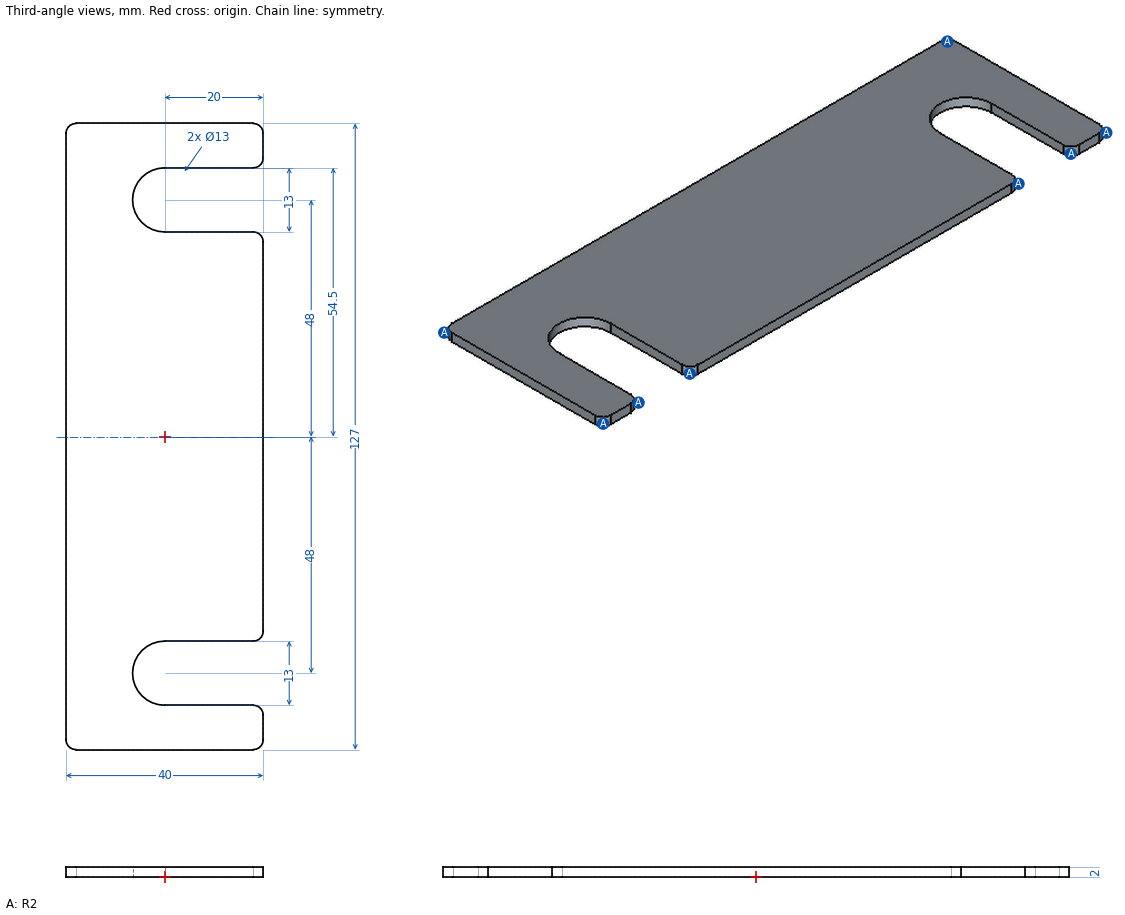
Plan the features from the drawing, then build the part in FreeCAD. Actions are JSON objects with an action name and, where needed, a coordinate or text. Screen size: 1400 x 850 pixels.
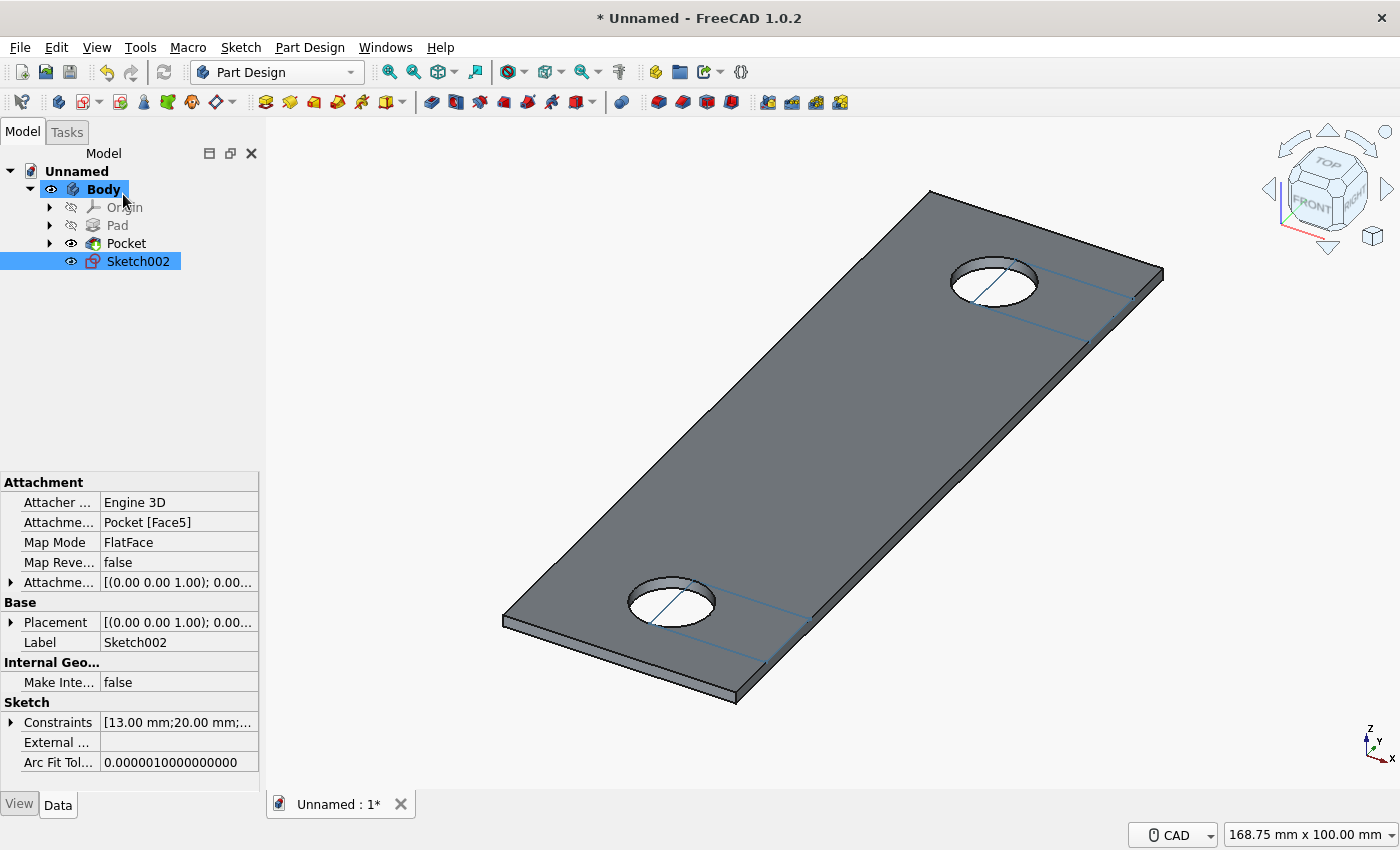
{"action": "left_click", "coordinate": [432, 102]}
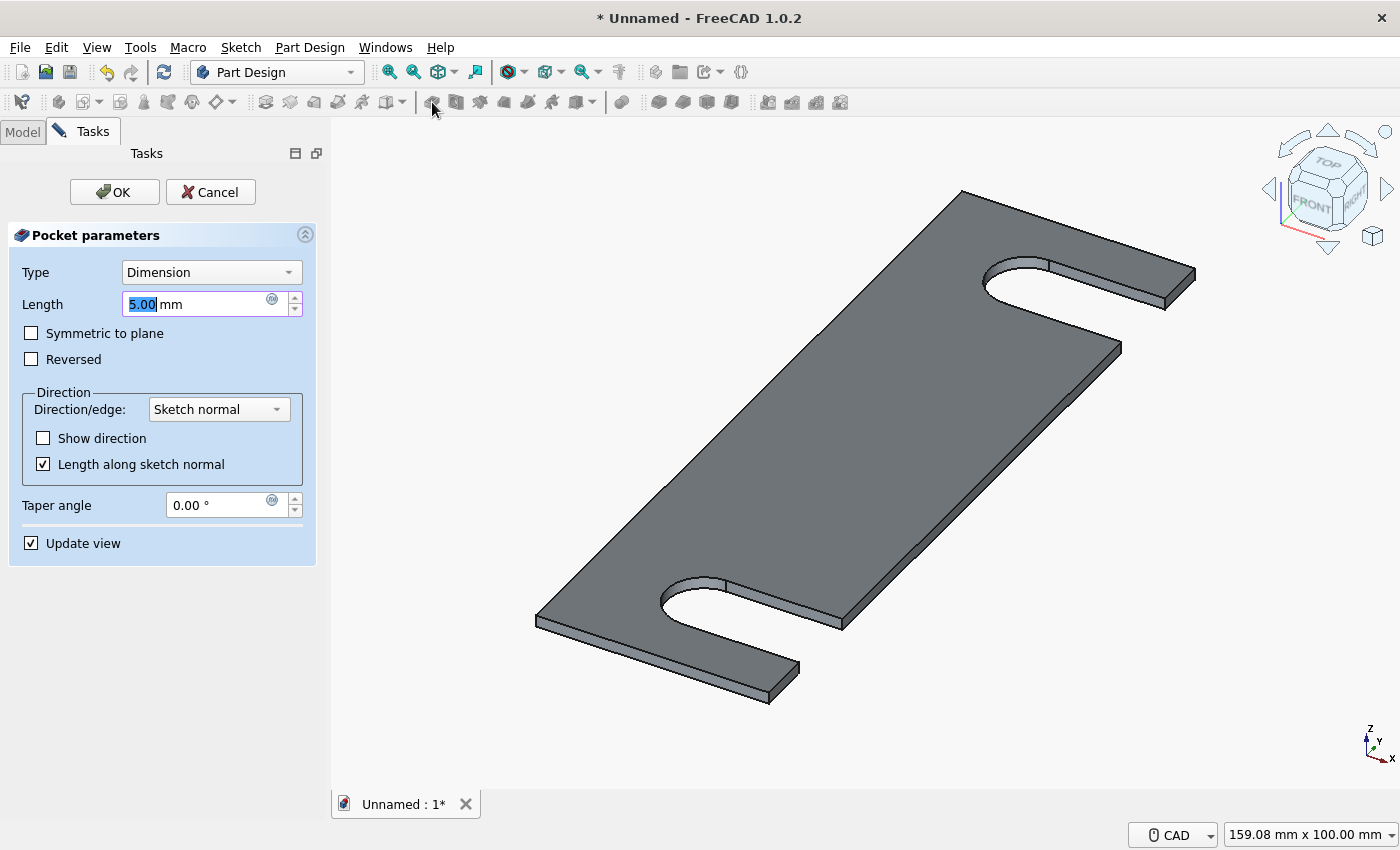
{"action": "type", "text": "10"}
{"action": "key", "text": "Tab"}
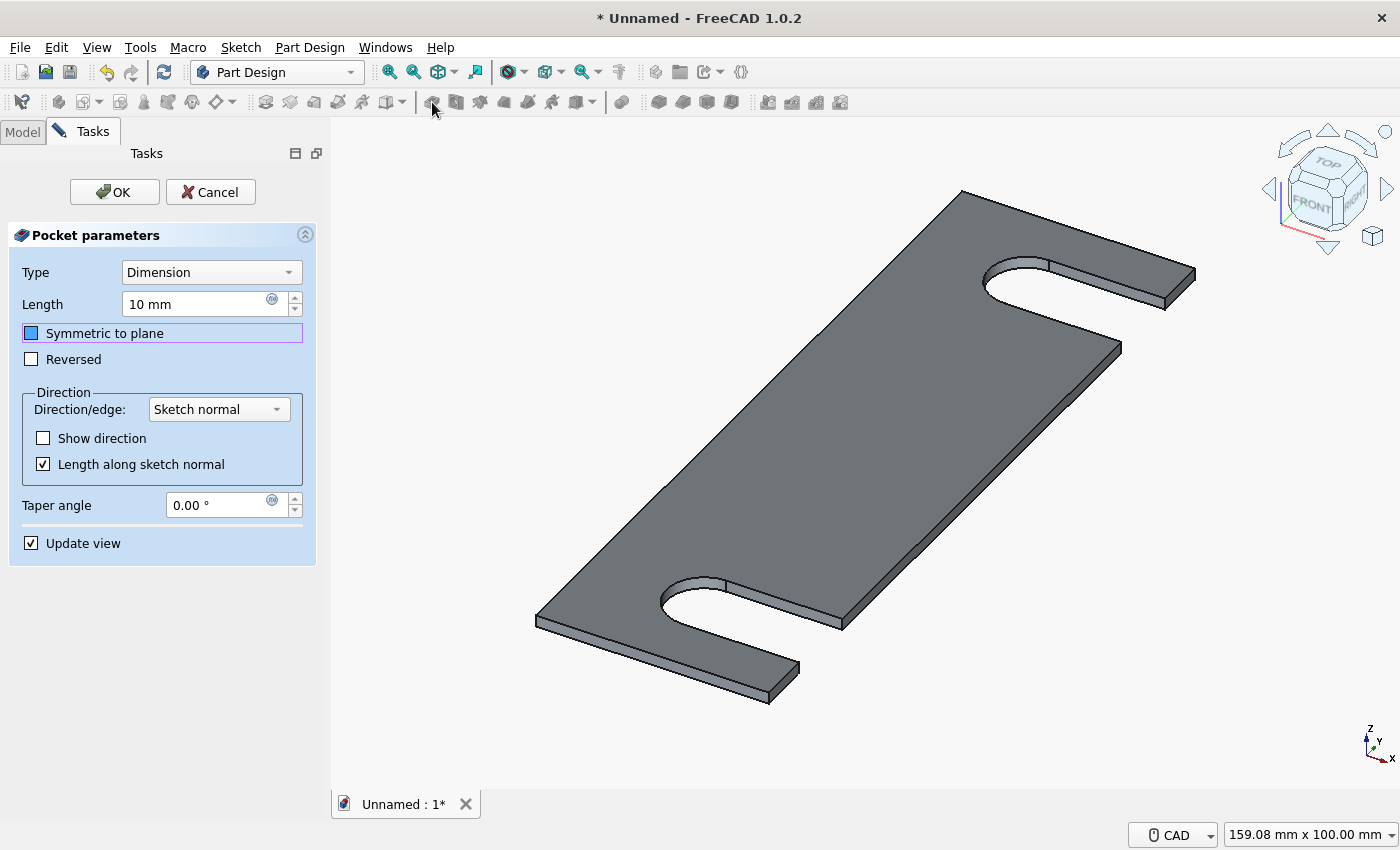
{"action": "left_click", "coordinate": [115, 192]}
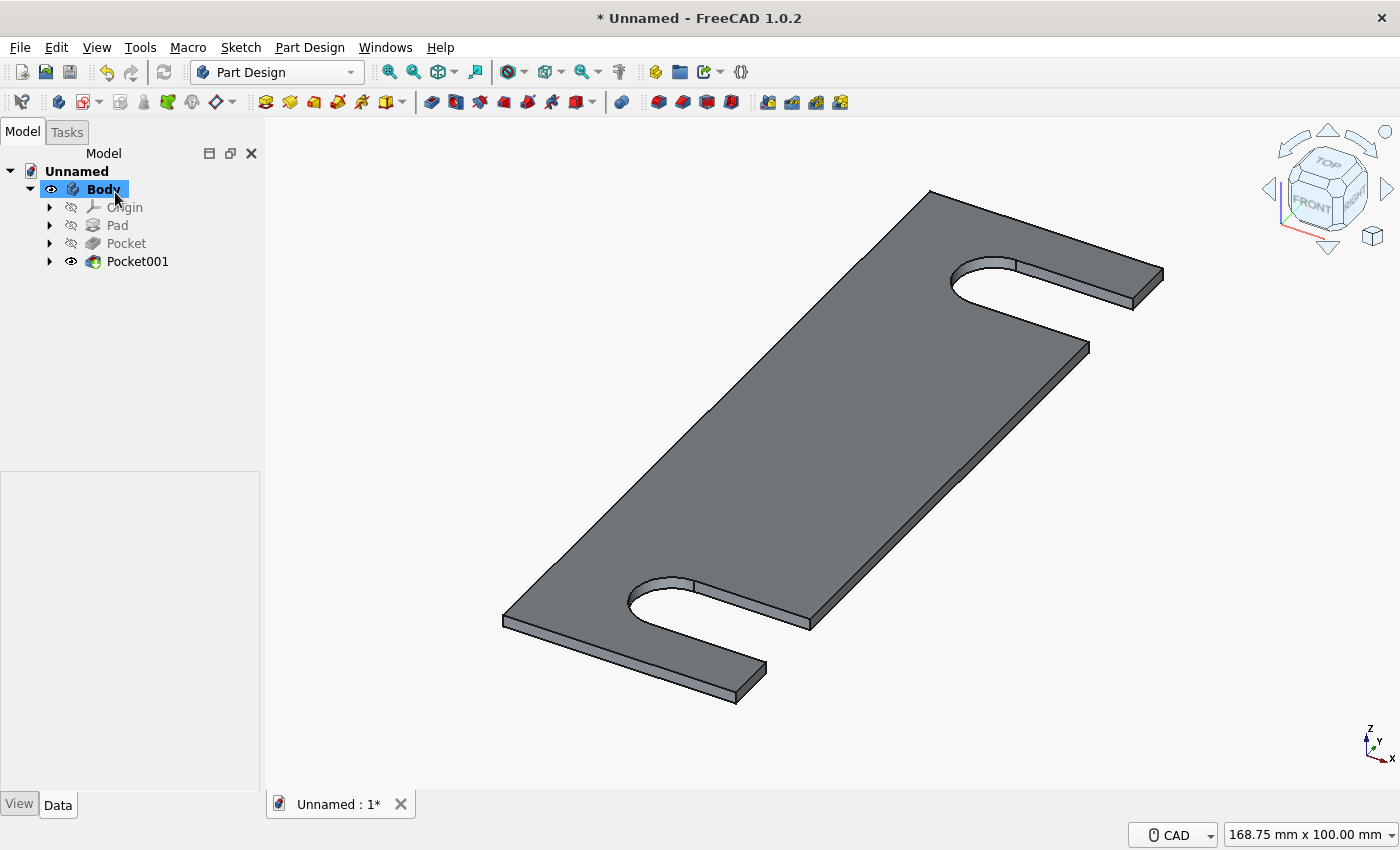
{"action": "left_click", "coordinate": [1133, 304]}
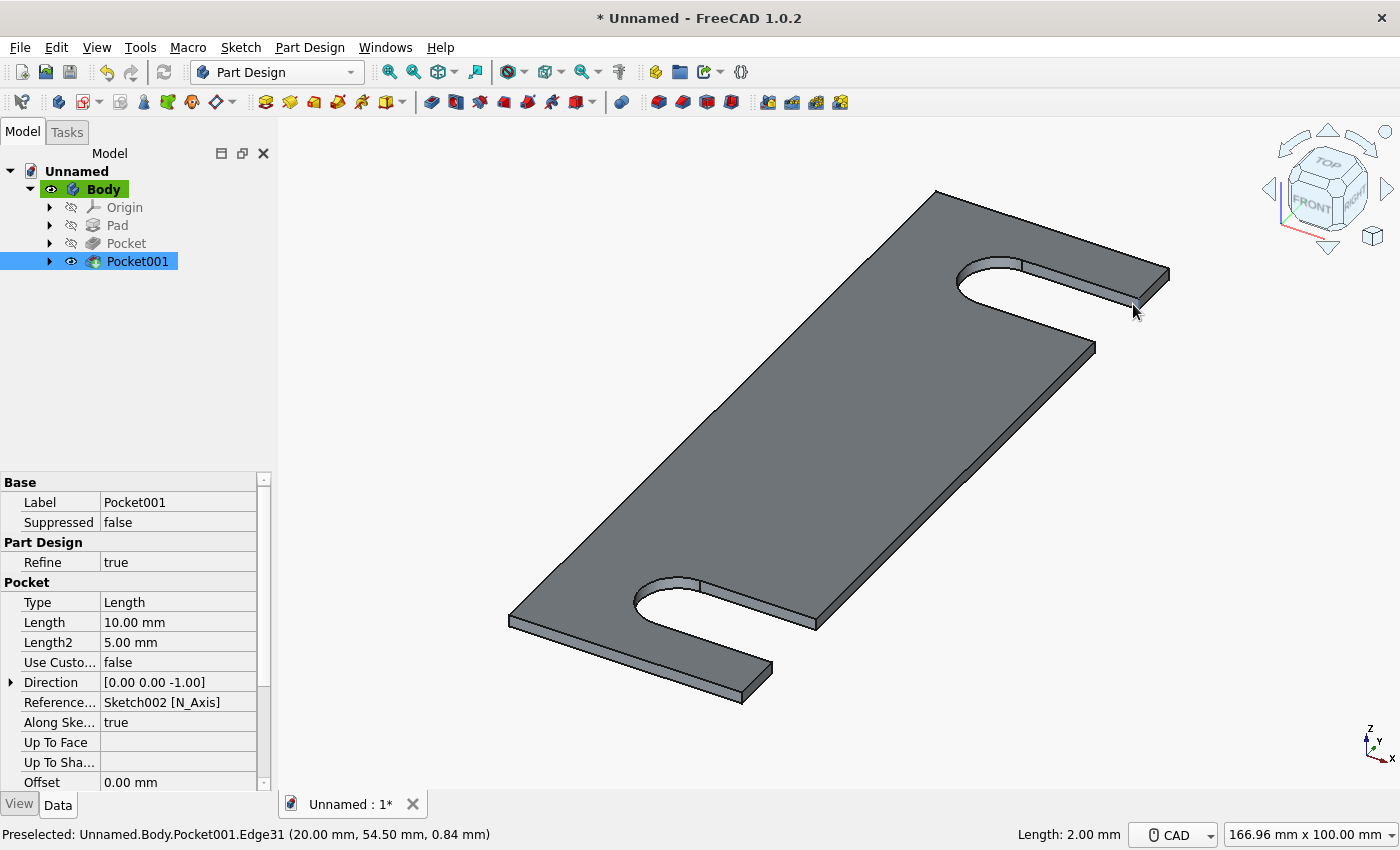
{"action": "left_click", "coordinate": [816, 624], "text": "ctrl"}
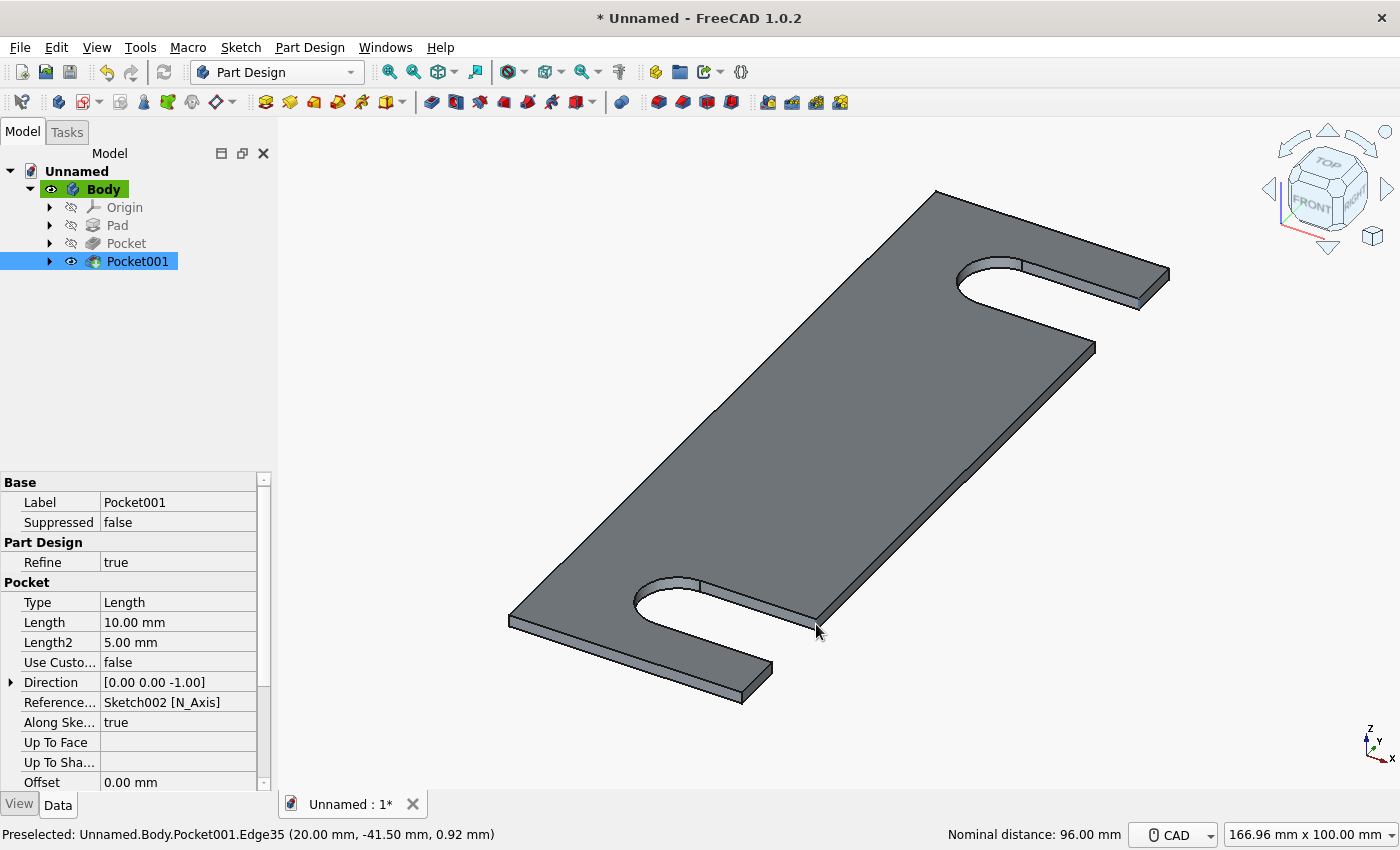
{"action": "left_click", "coordinate": [742, 698], "text": "ctrl"}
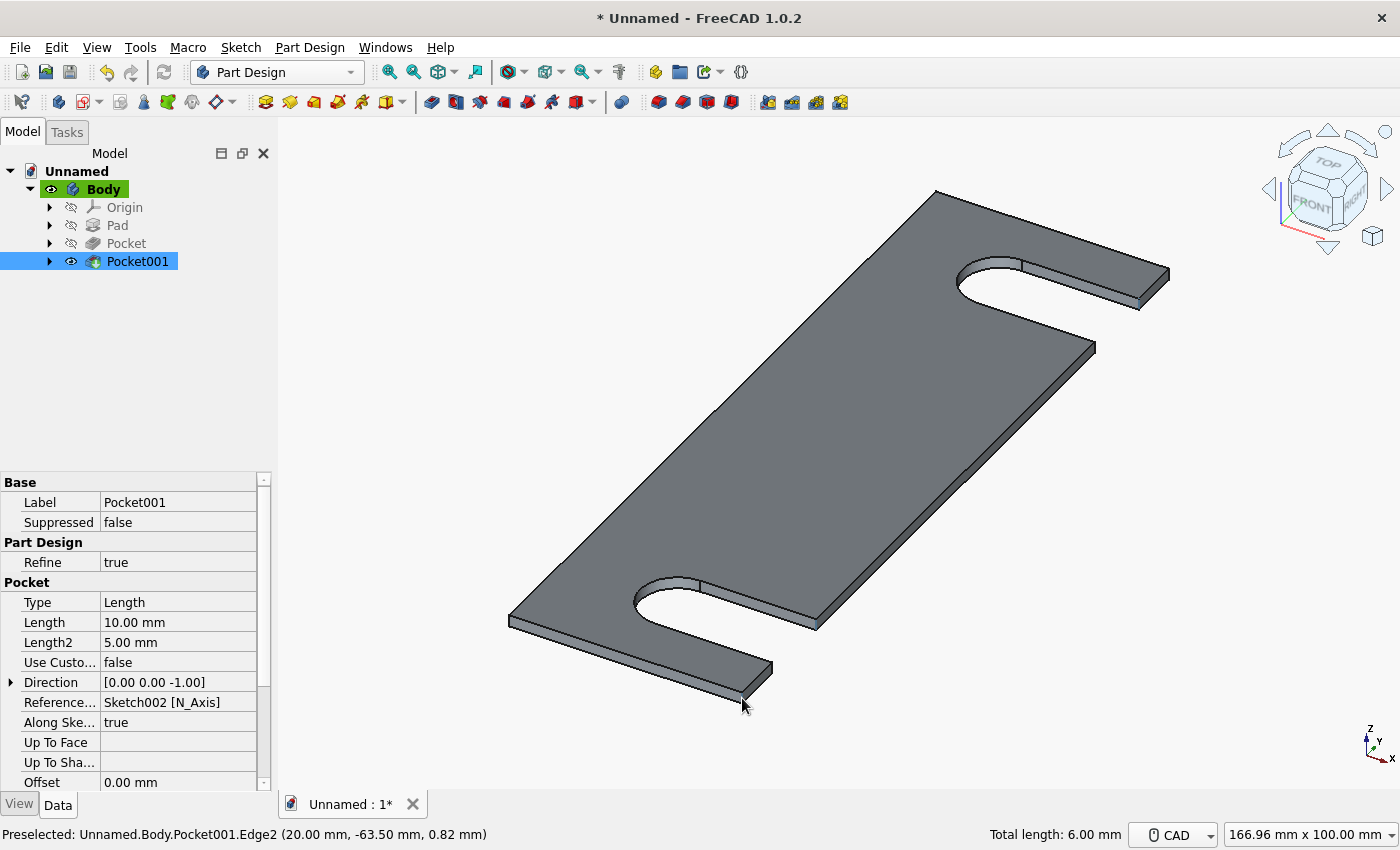
{"action": "scroll", "coordinate": [1095, 347], "scroll_direction": "up", "scroll_amount": 6}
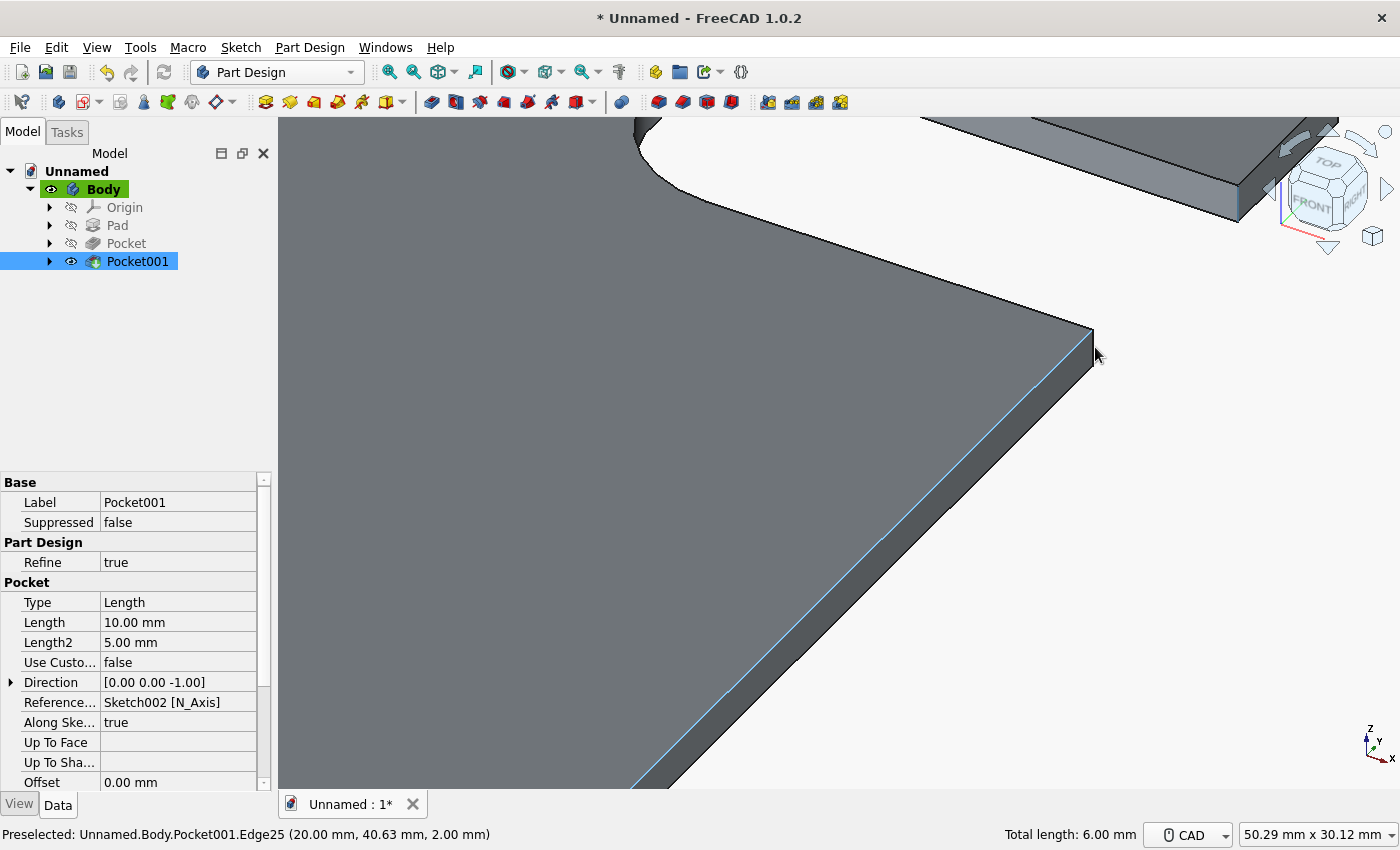
{"action": "key", "text": "v f"}